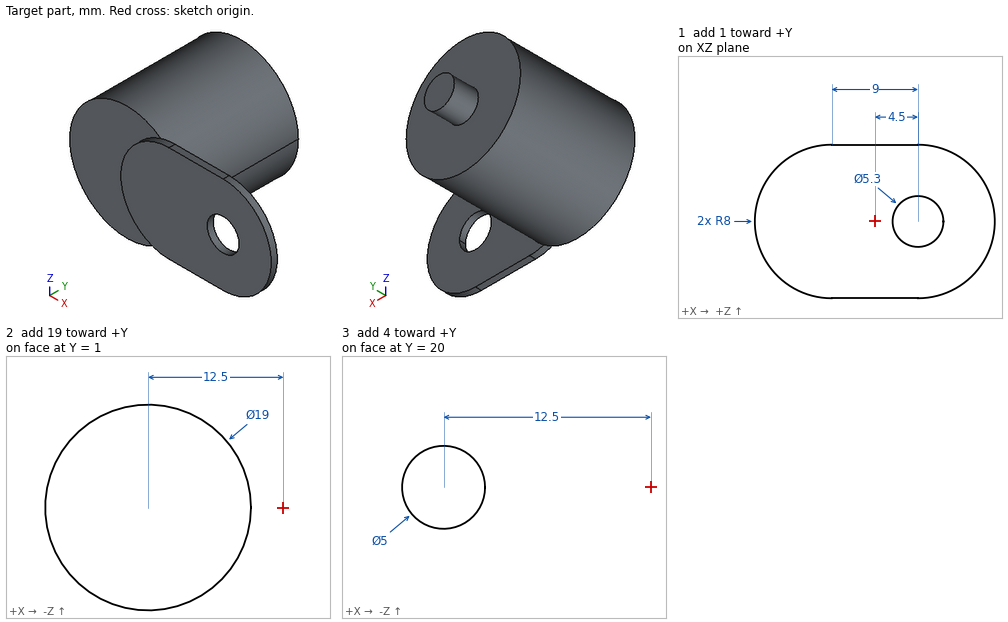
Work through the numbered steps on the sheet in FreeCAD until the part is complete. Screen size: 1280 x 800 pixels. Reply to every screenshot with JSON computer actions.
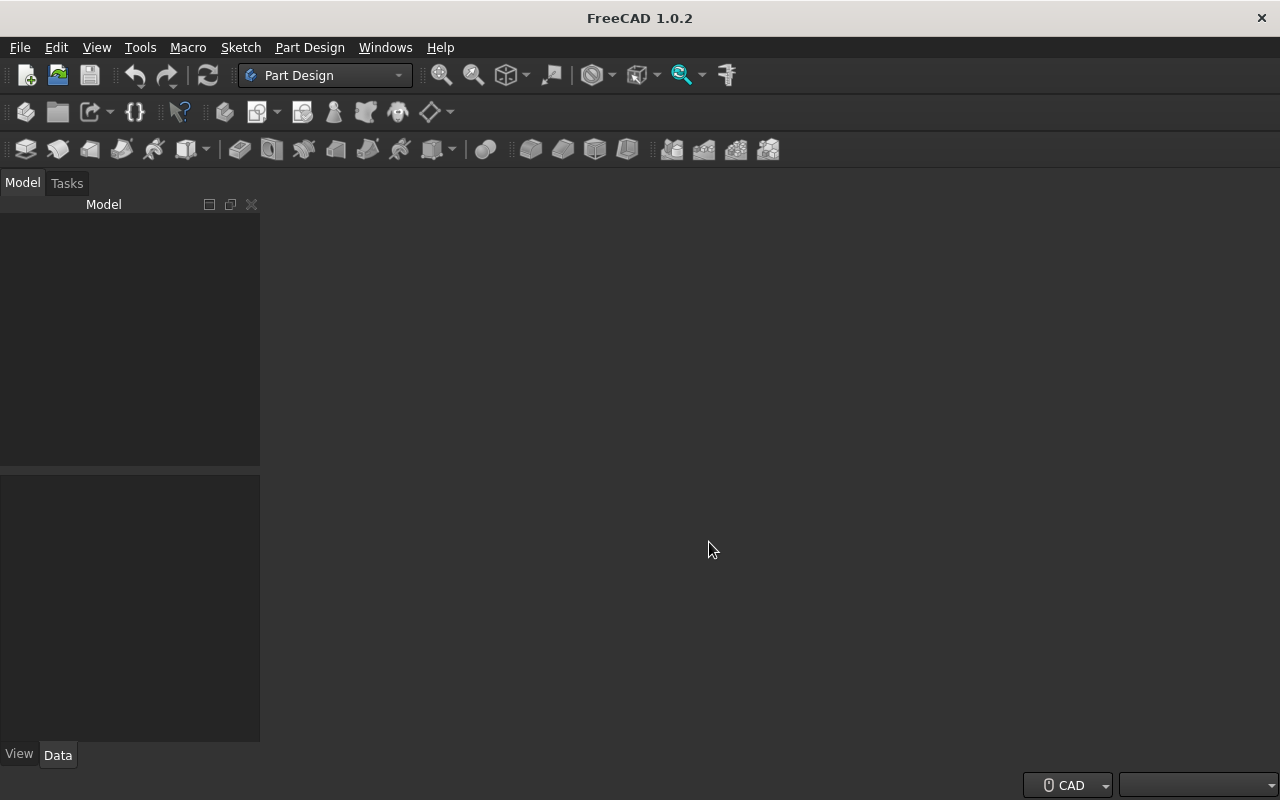
{"action": "left_click", "coordinate": [26, 76]}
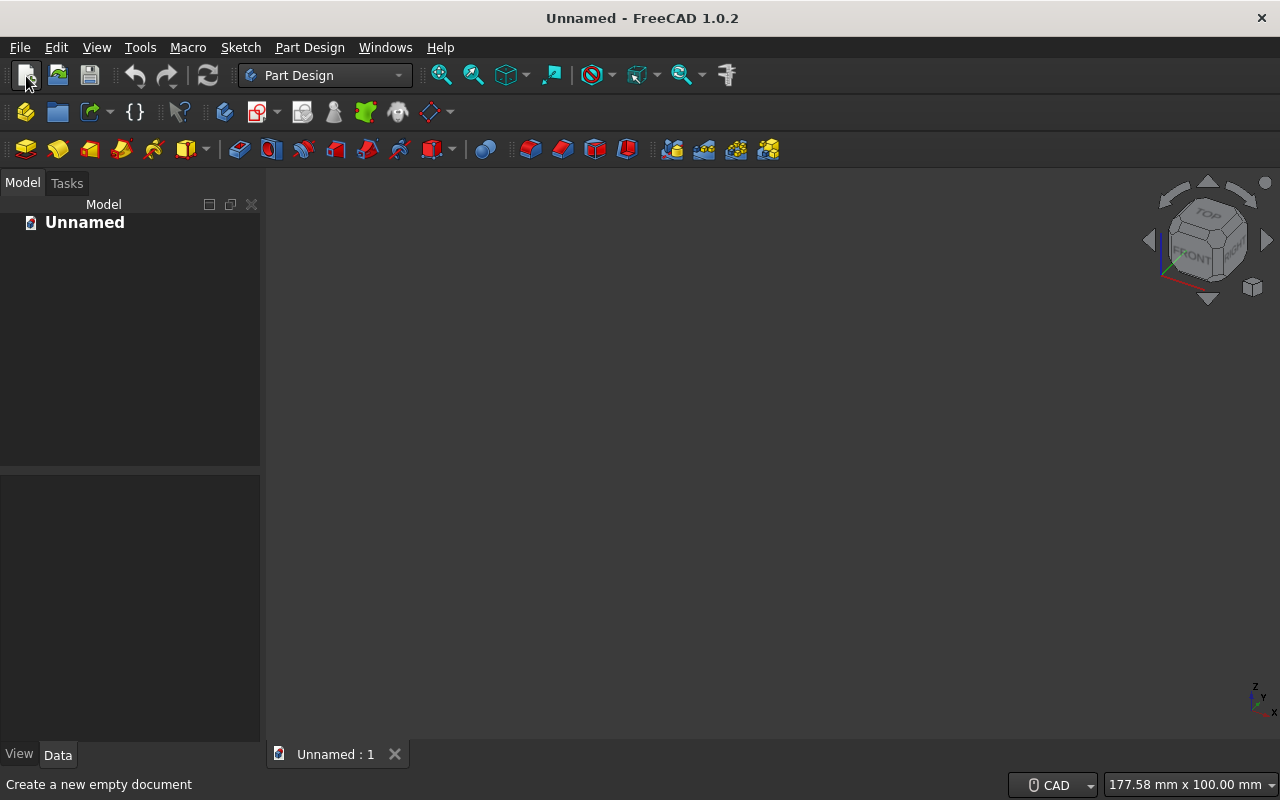
{"action": "left_click", "coordinate": [258, 112]}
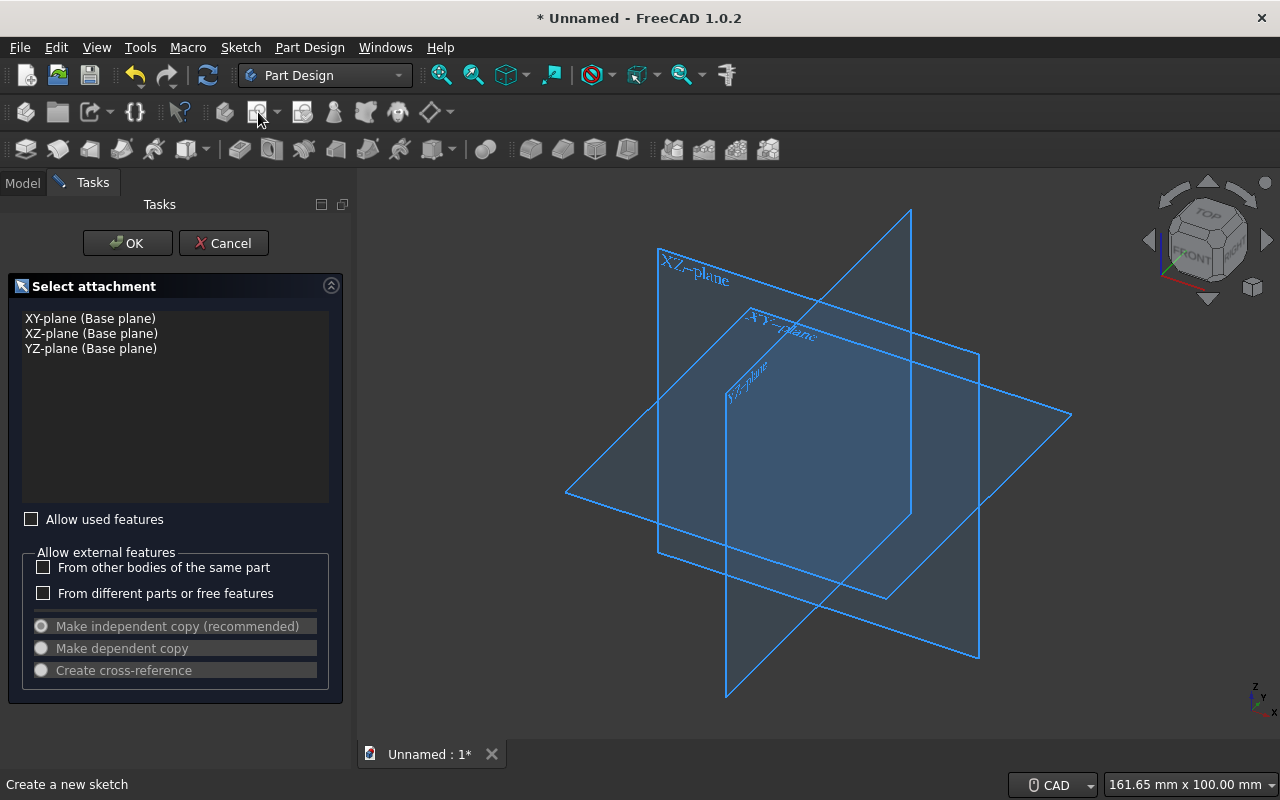
{"action": "left_click", "coordinate": [82, 334]}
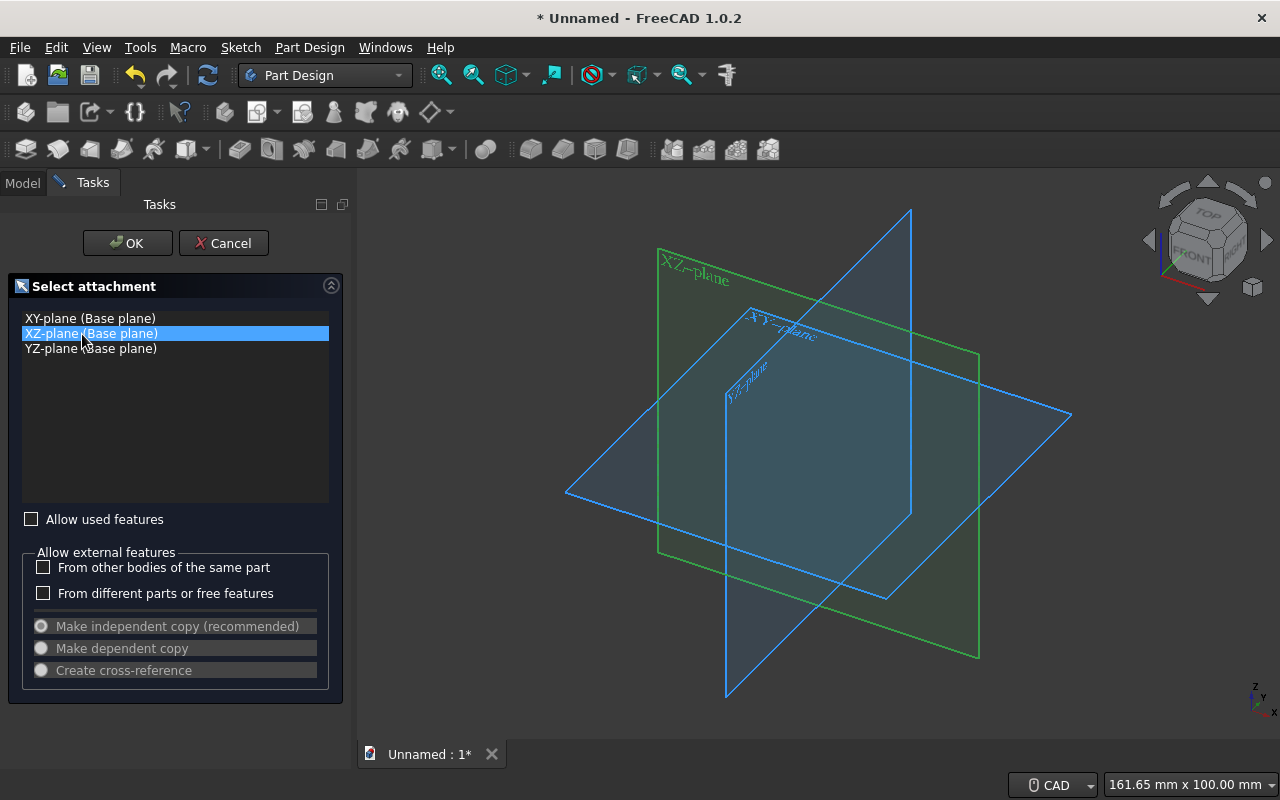
{"action": "left_click", "coordinate": [128, 243]}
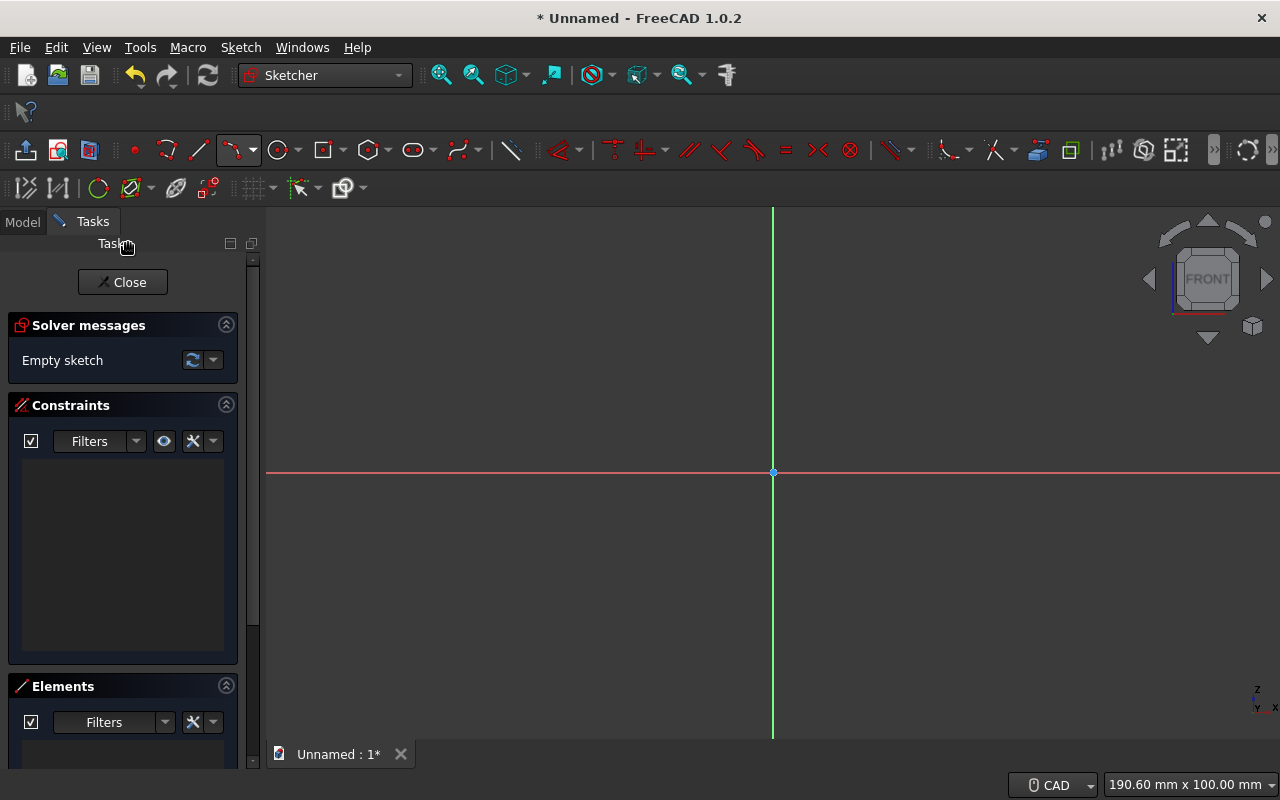
{"action": "scroll", "coordinate": [795, 473], "scroll_direction": "up", "scroll_amount": 7}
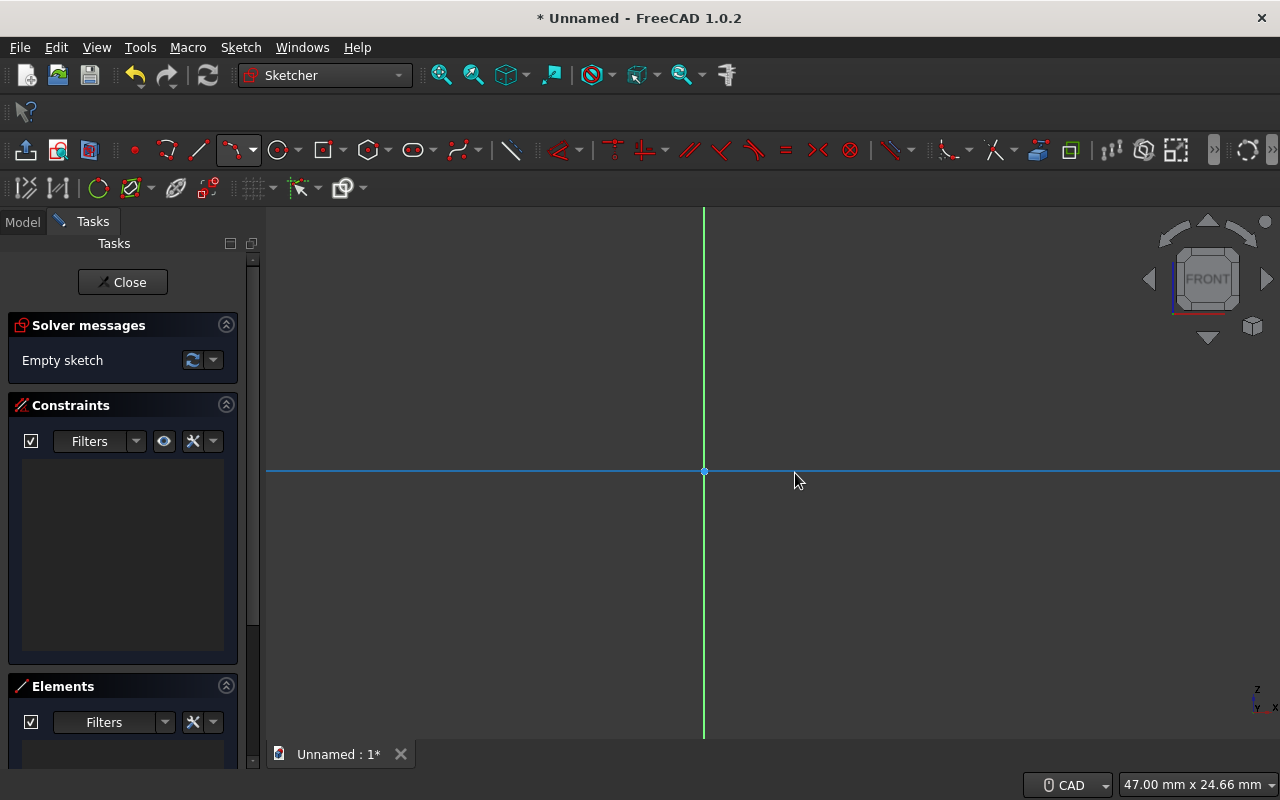
{"action": "left_click", "coordinate": [414, 150]}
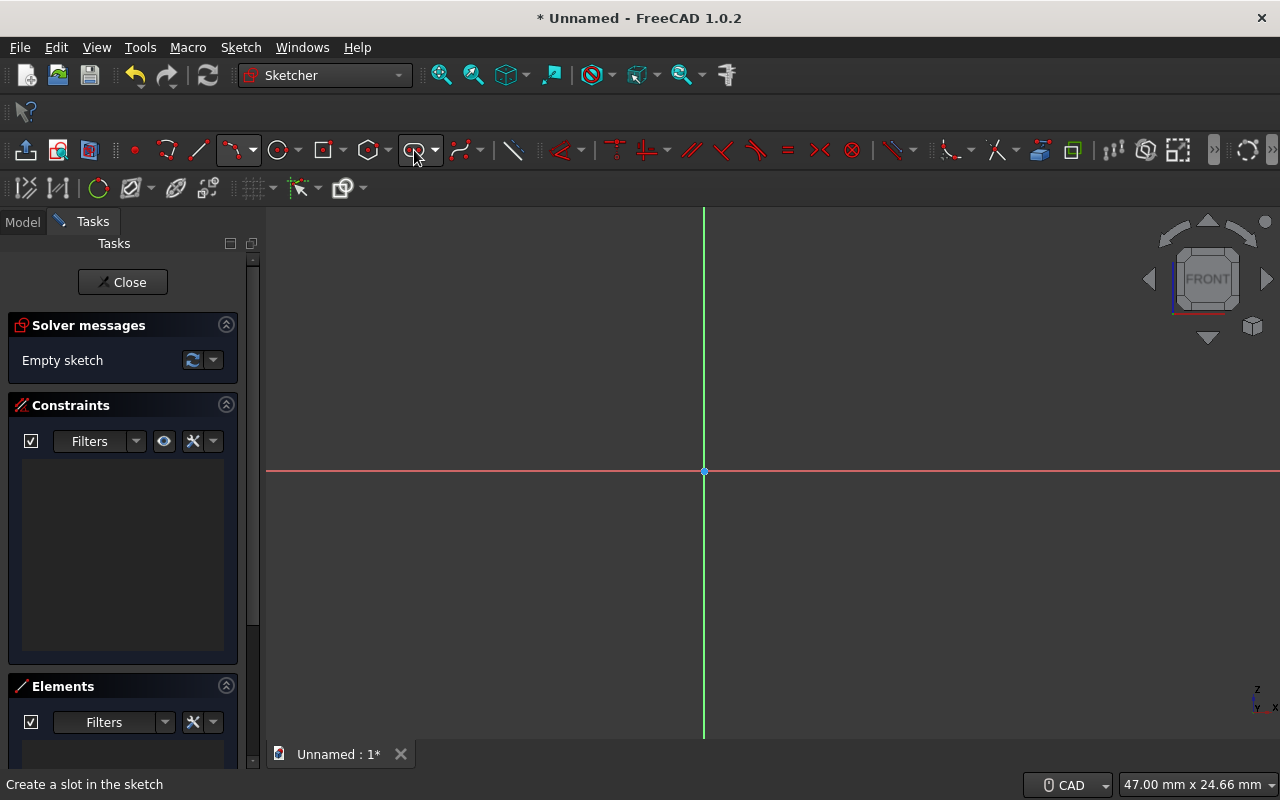
{"action": "left_click", "coordinate": [607, 471]}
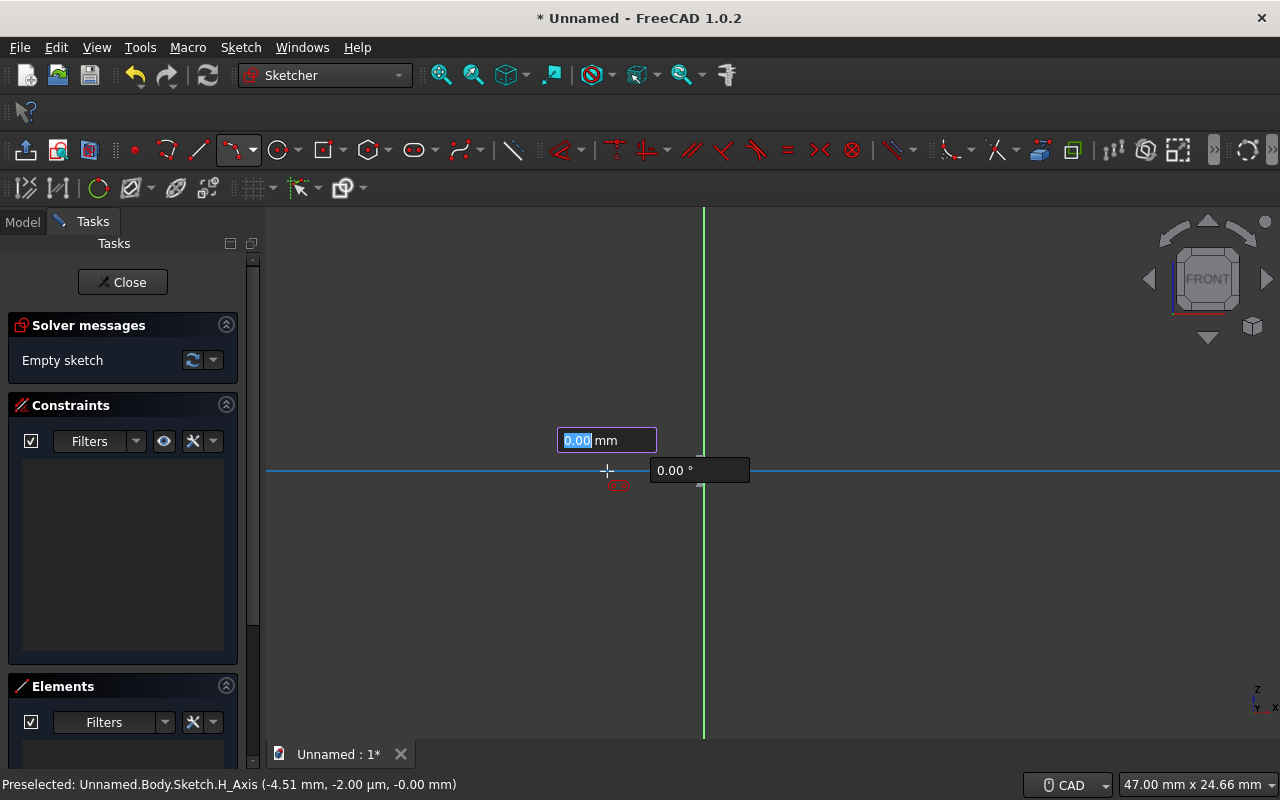
{"action": "left_click", "coordinate": [801, 462]}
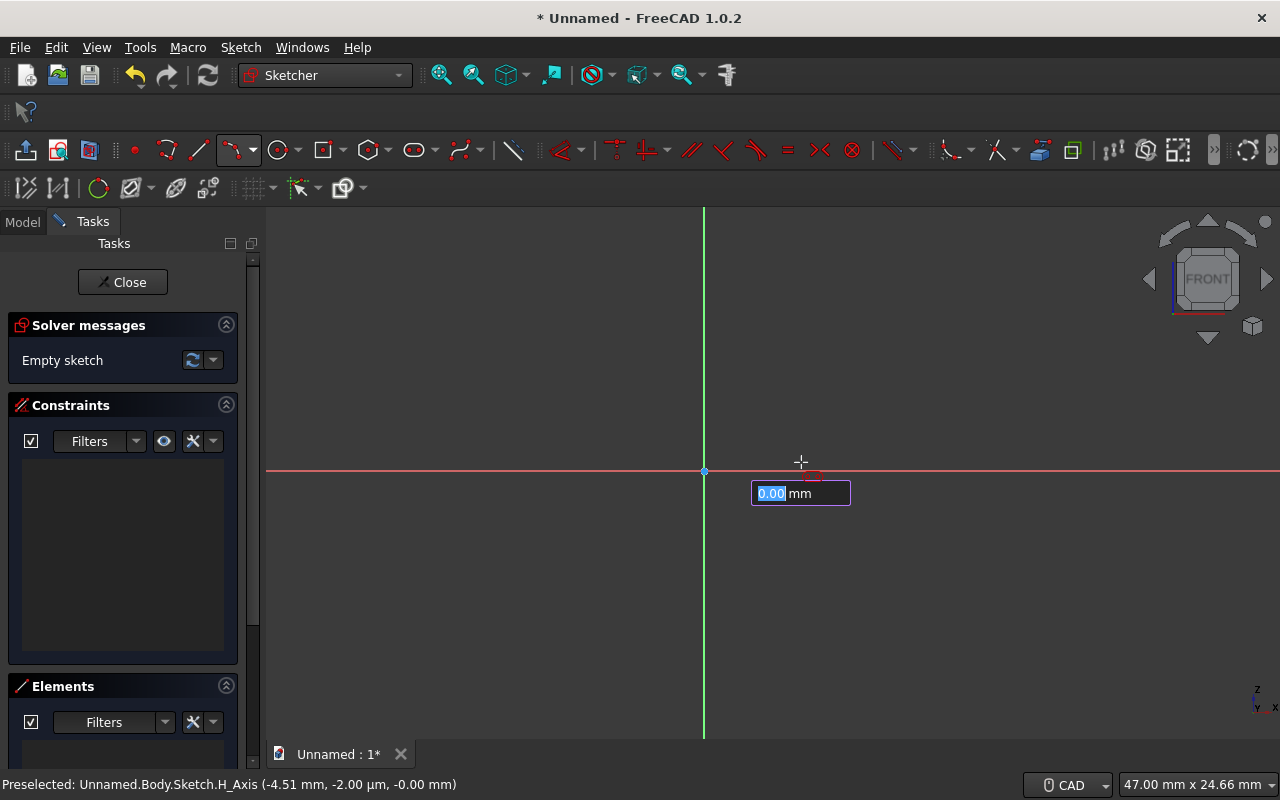
{"action": "left_click", "coordinate": [733, 644]}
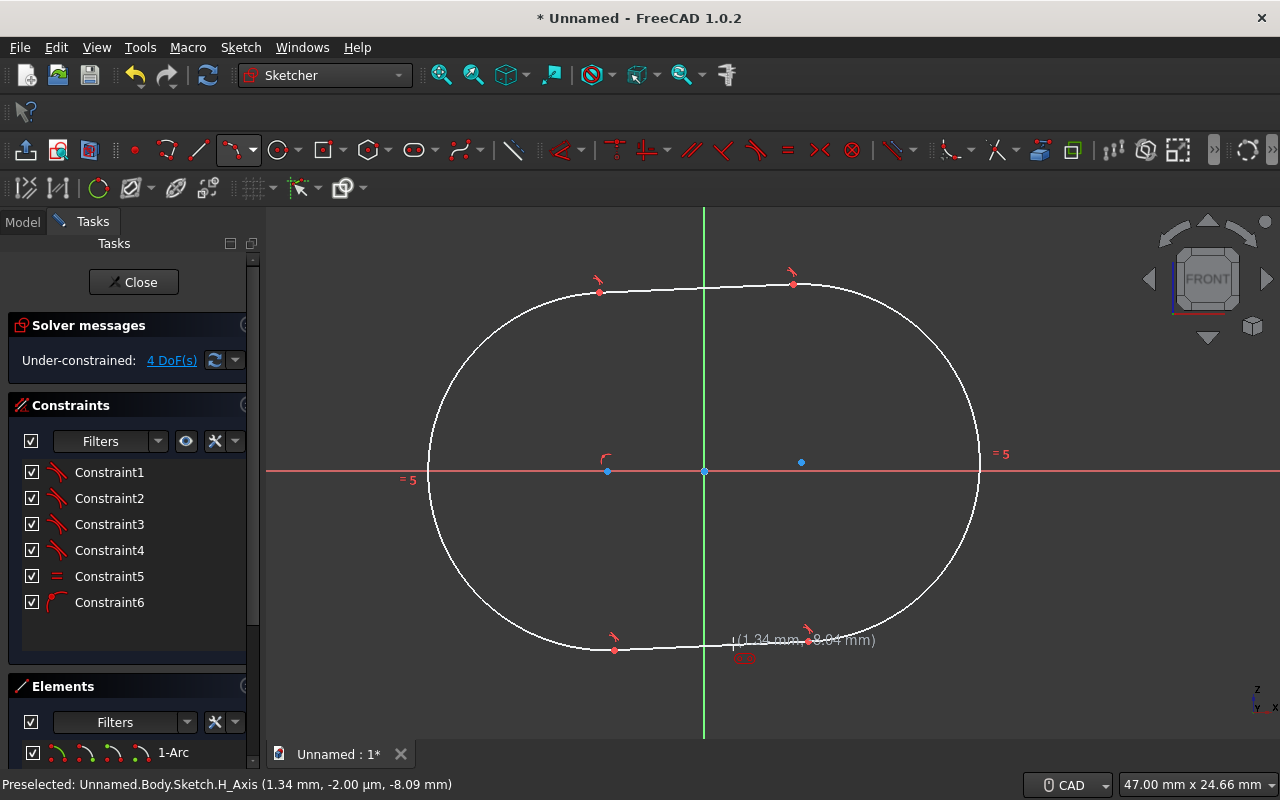
{"action": "left_click", "coordinate": [278, 150]}